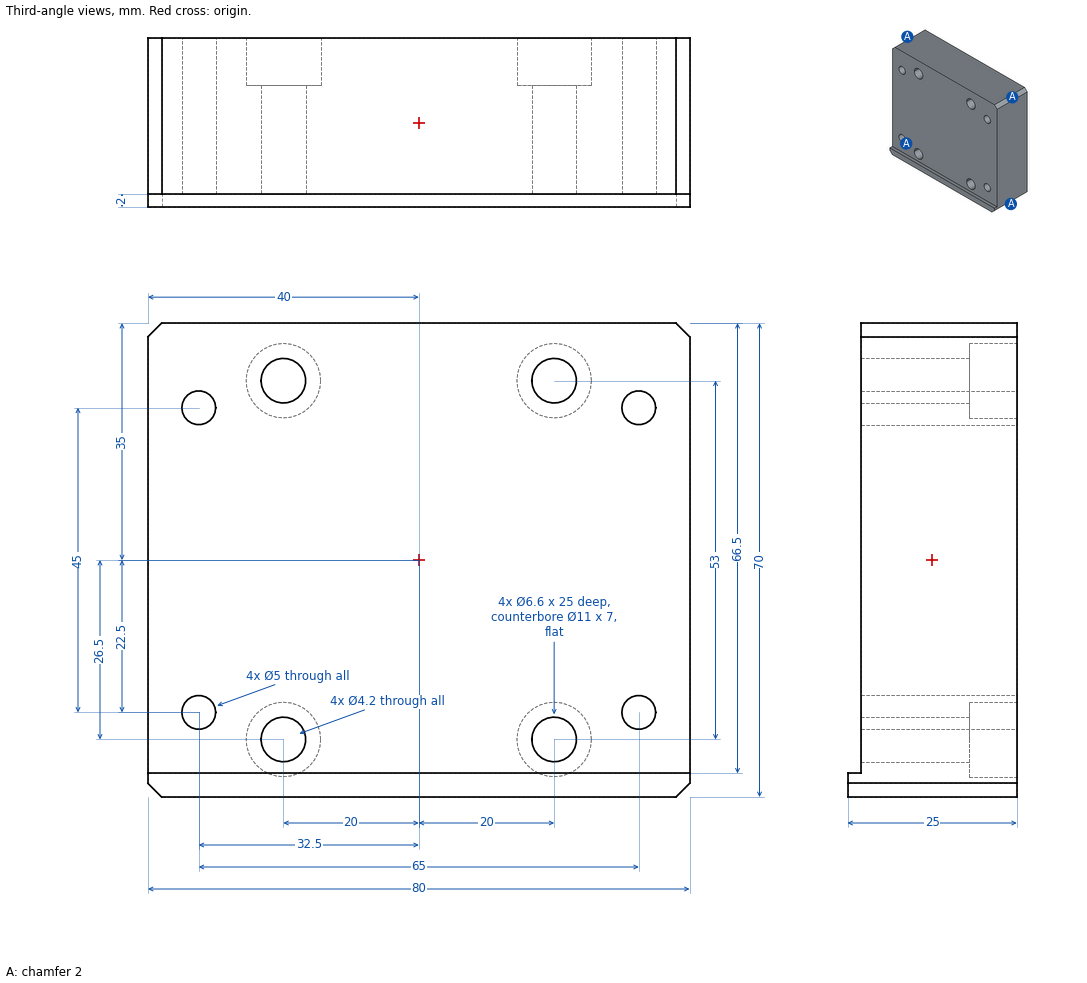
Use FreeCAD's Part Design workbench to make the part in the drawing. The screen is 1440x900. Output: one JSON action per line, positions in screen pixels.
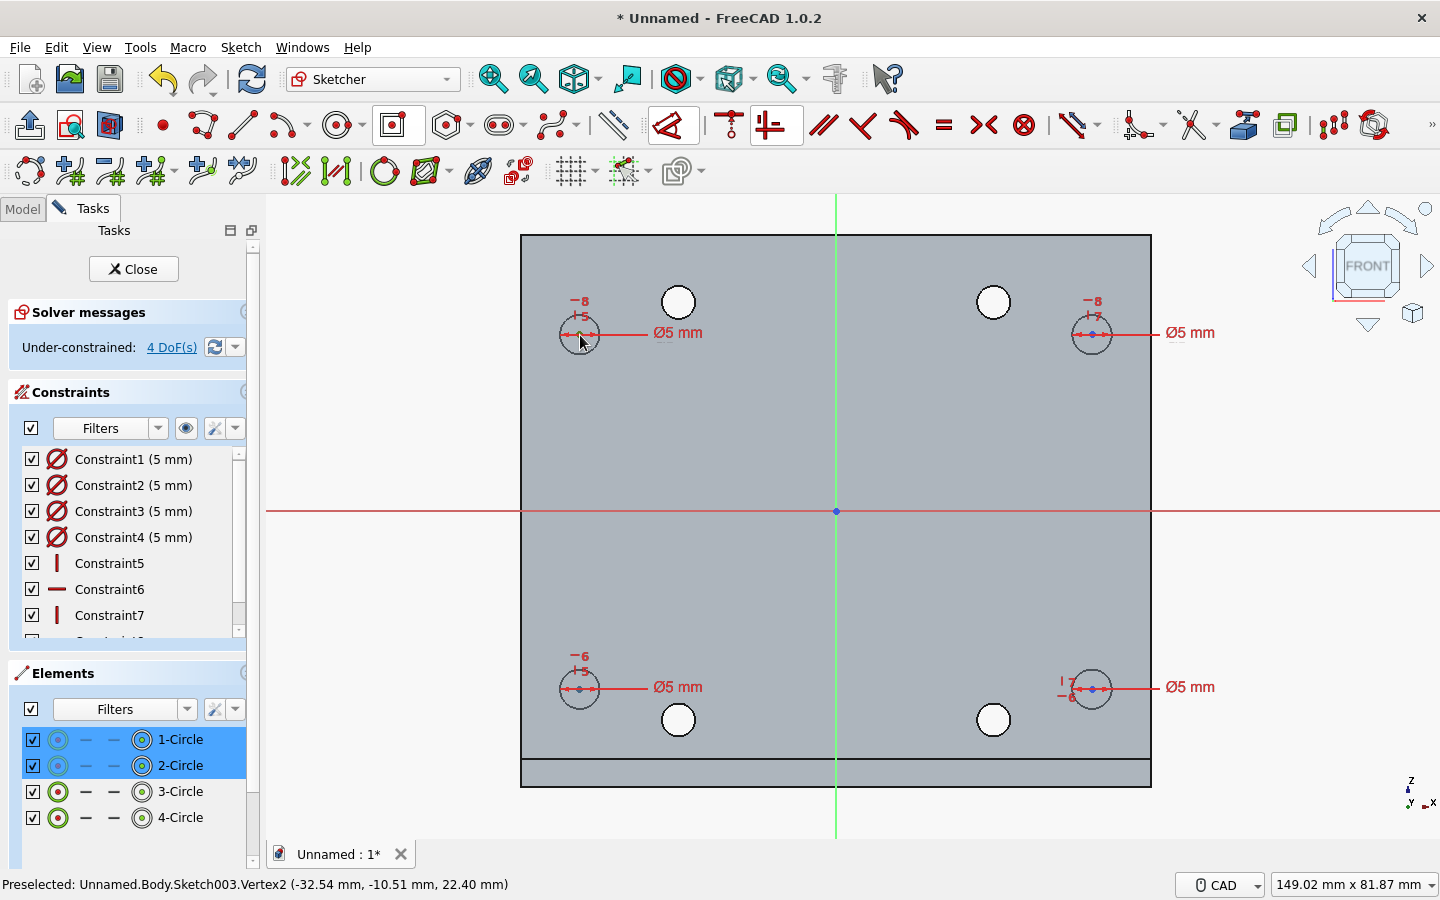
{"action": "left_click", "coordinate": [694, 126]}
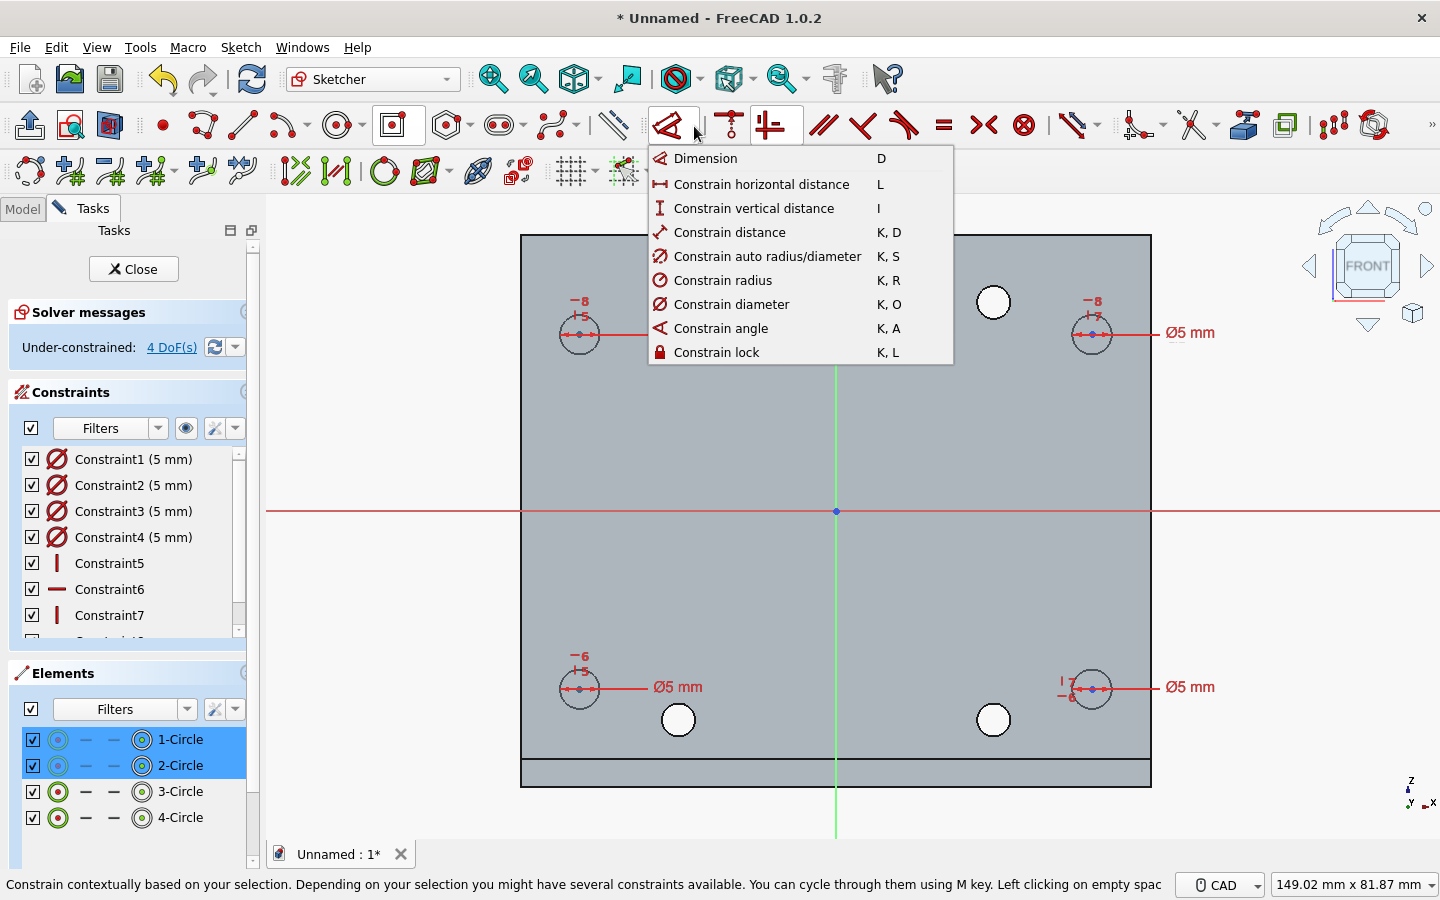
{"action": "left_click", "coordinate": [801, 208]}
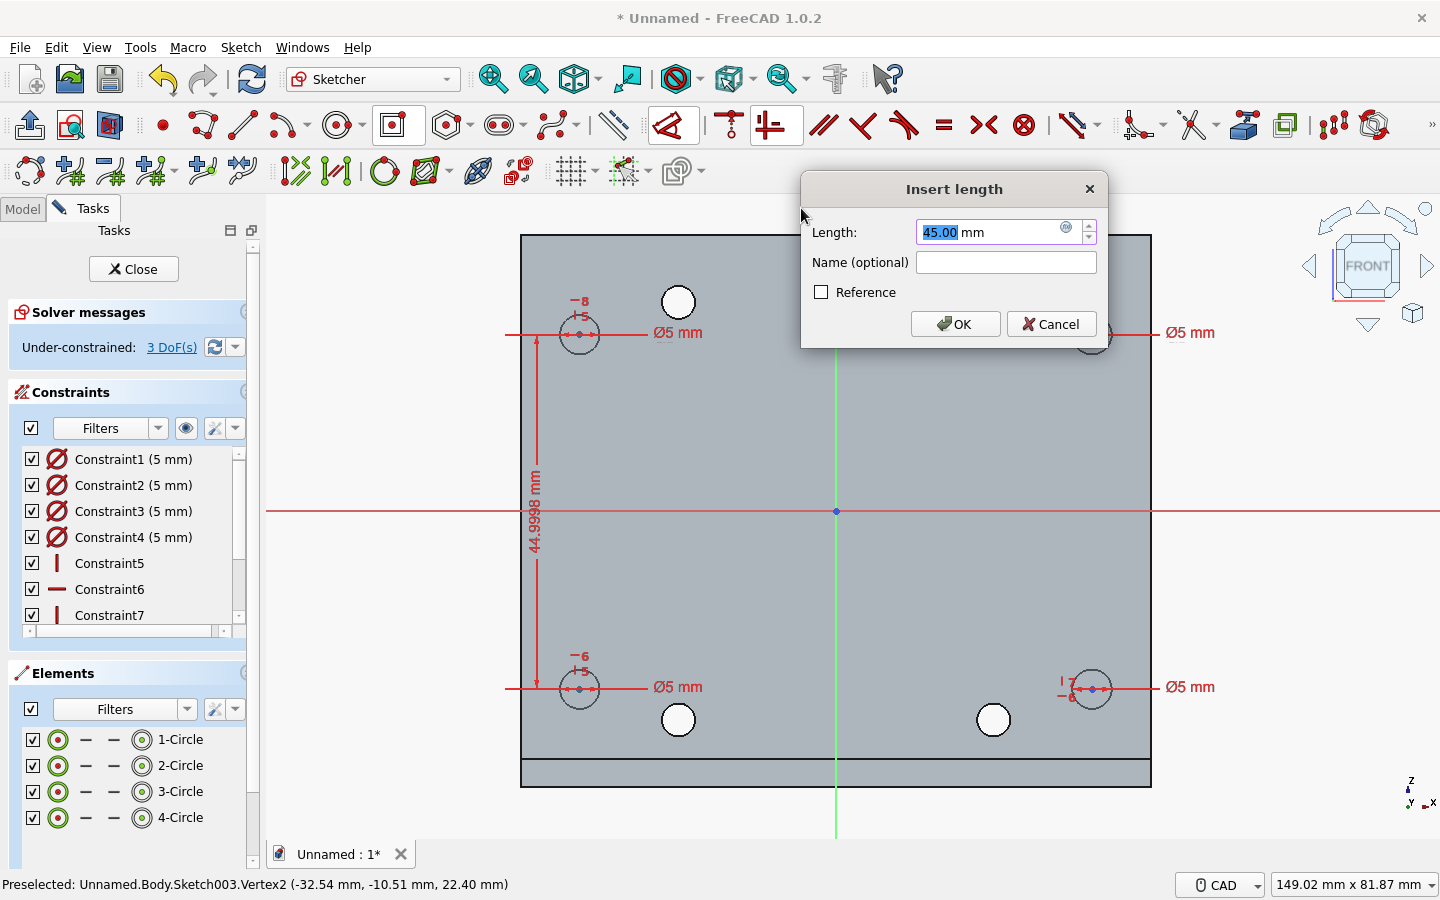
{"action": "type", "text": "45"}
{"action": "key", "text": "Return"}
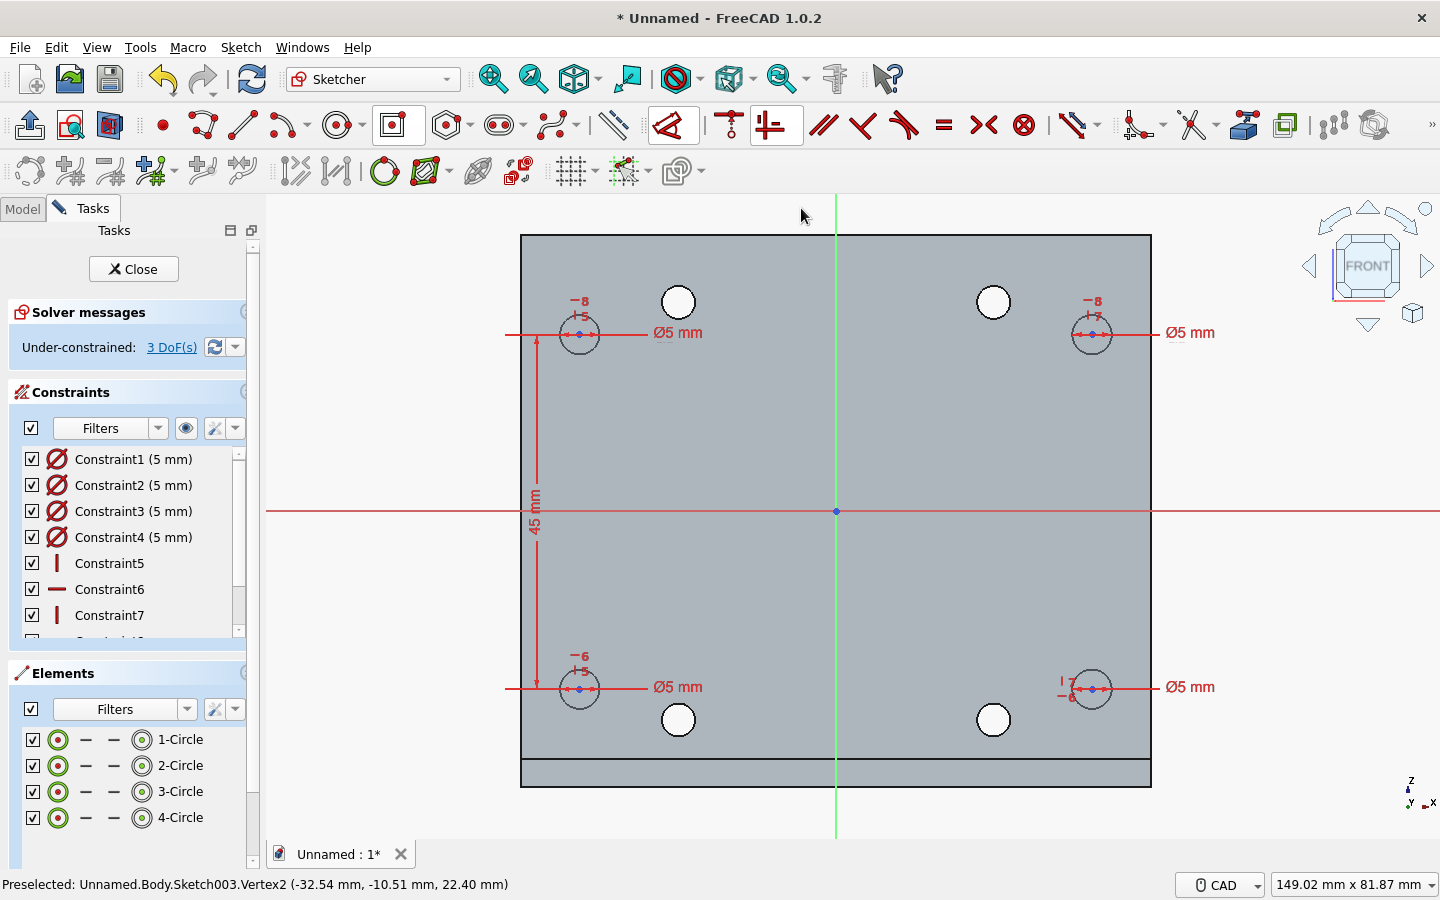
{"action": "left_click", "coordinate": [580, 689]}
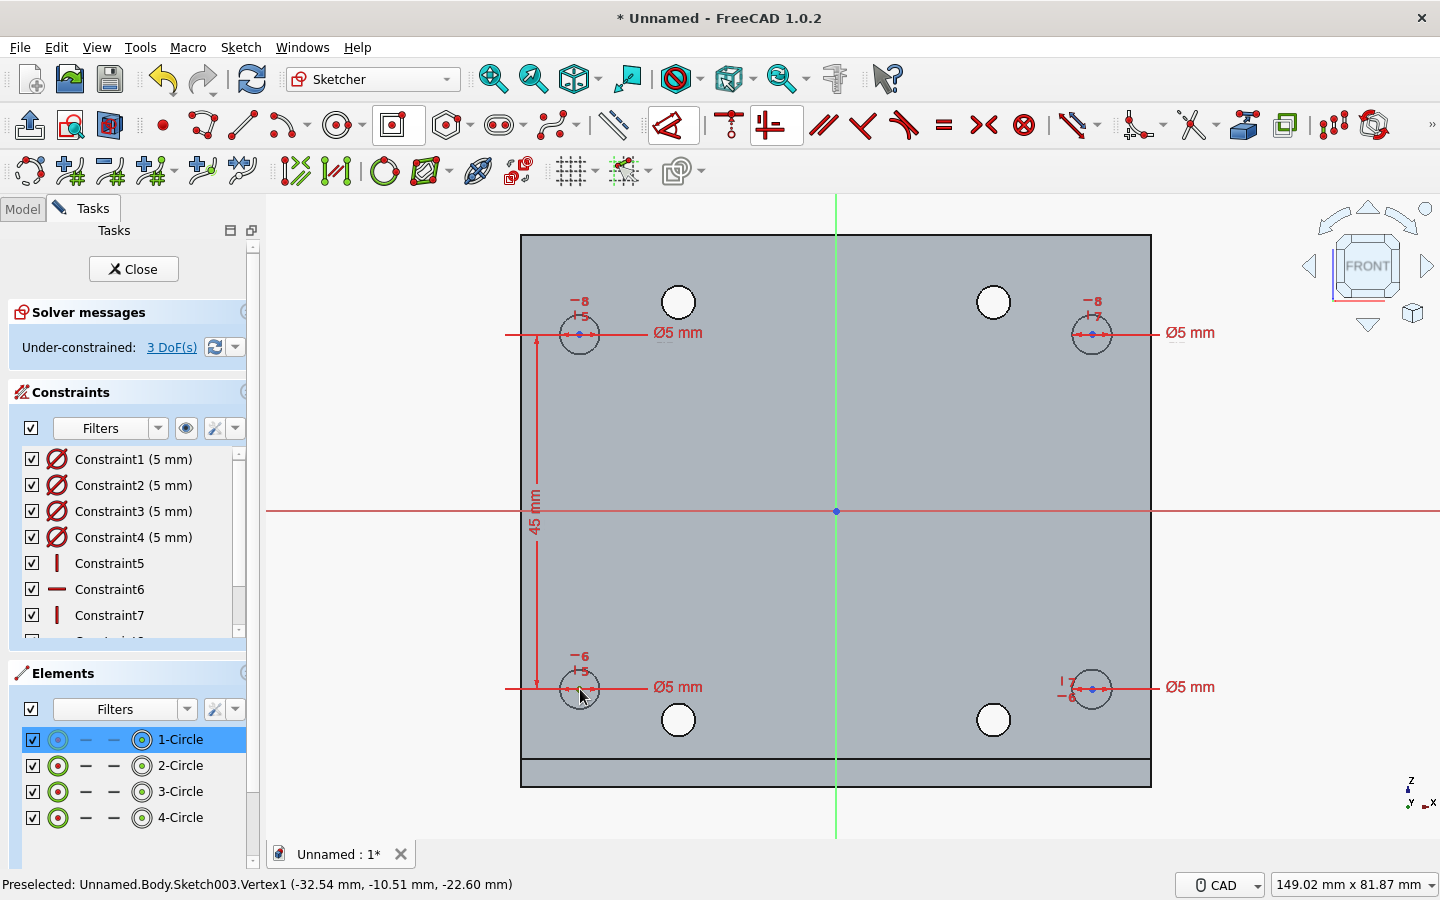
{"action": "left_click", "coordinate": [1092, 689]}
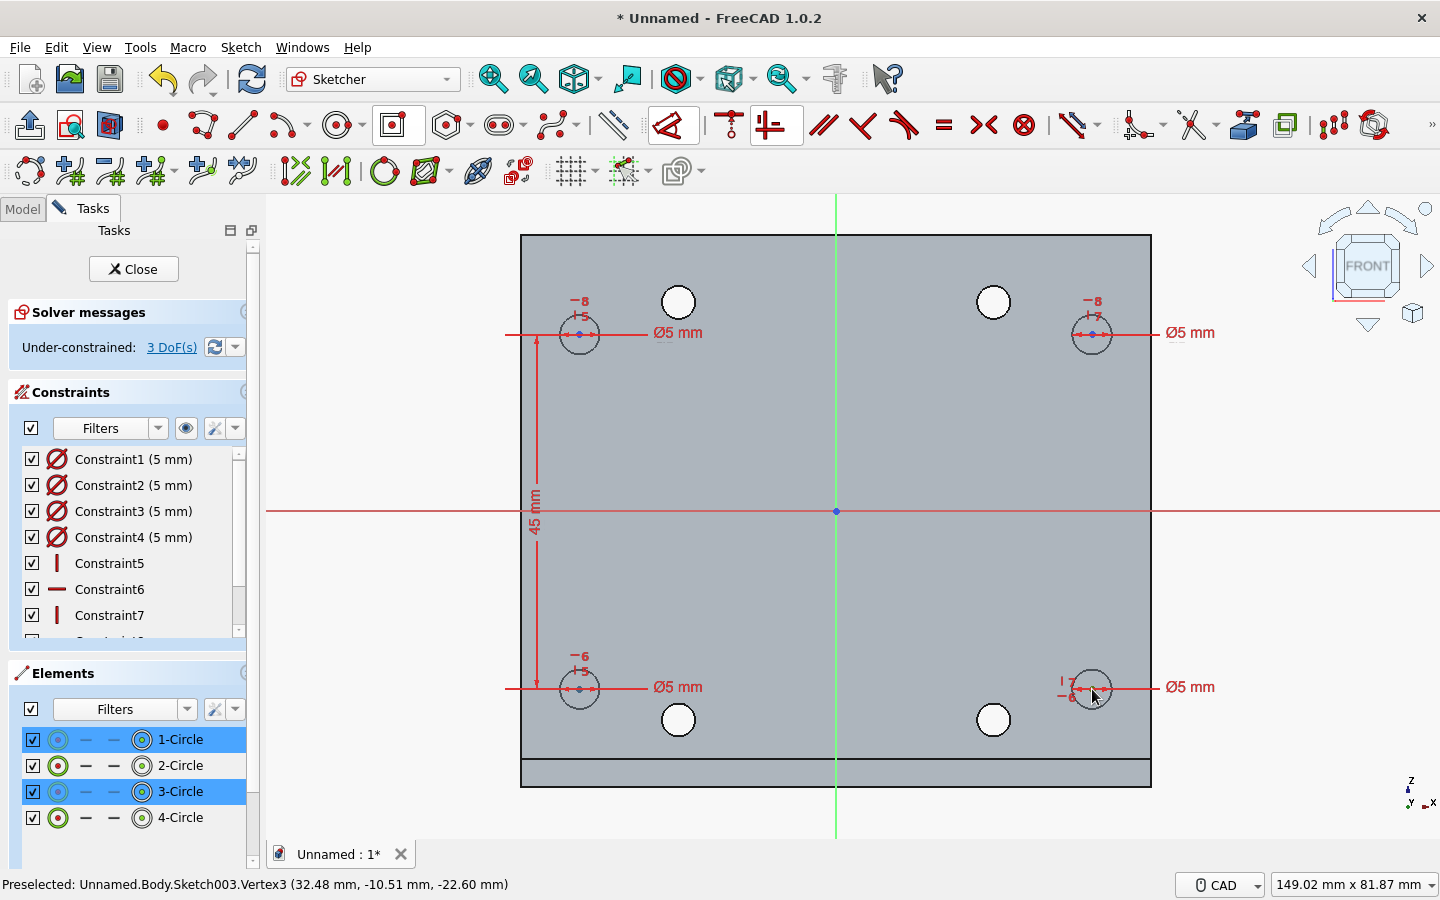
{"action": "key", "text": "l"}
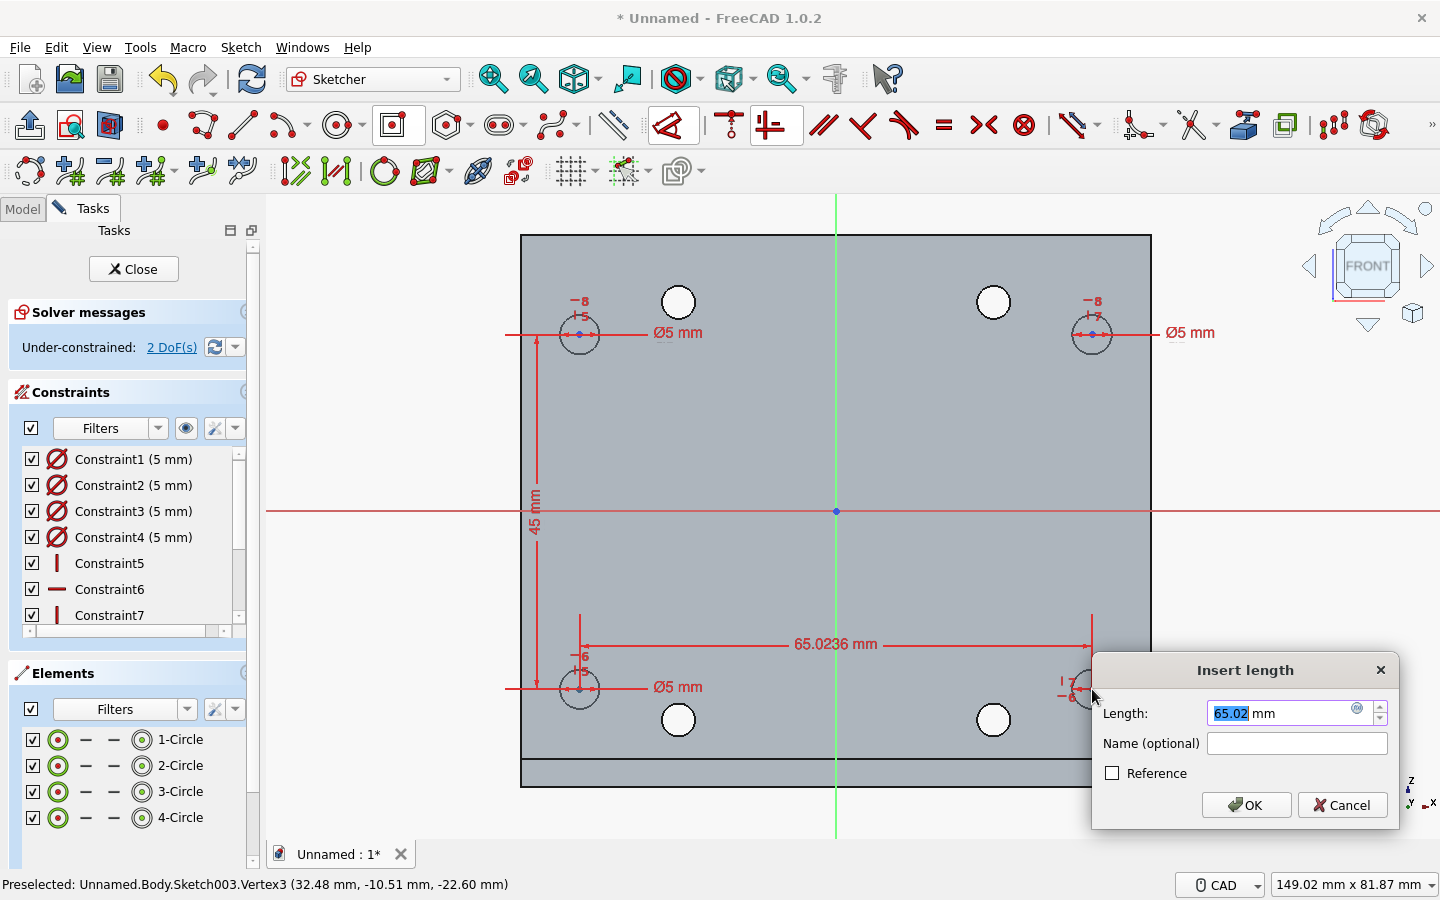
{"action": "type", "text": "65"}
{"action": "key", "text": "Return"}